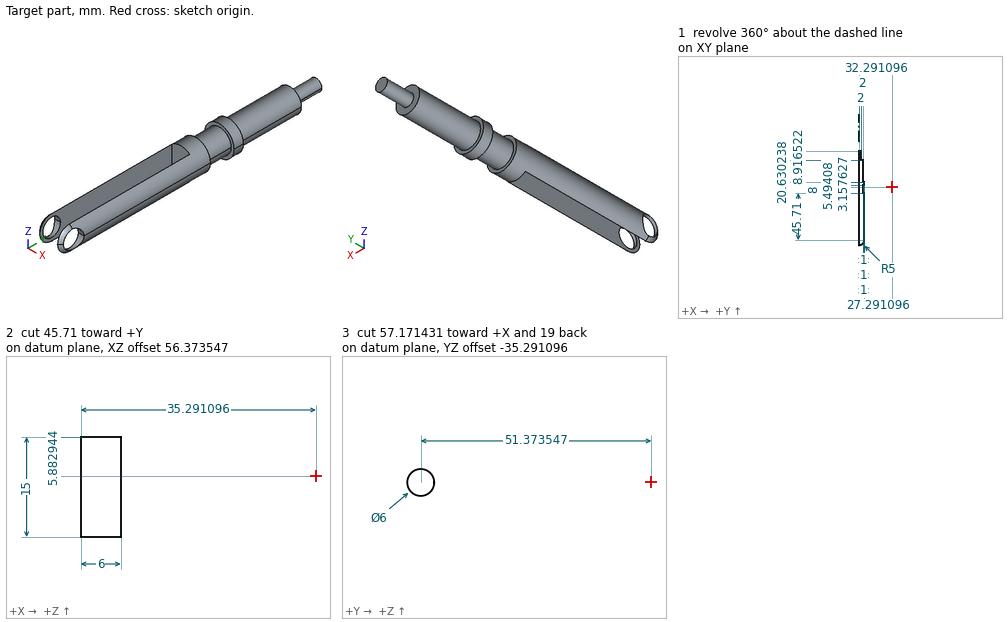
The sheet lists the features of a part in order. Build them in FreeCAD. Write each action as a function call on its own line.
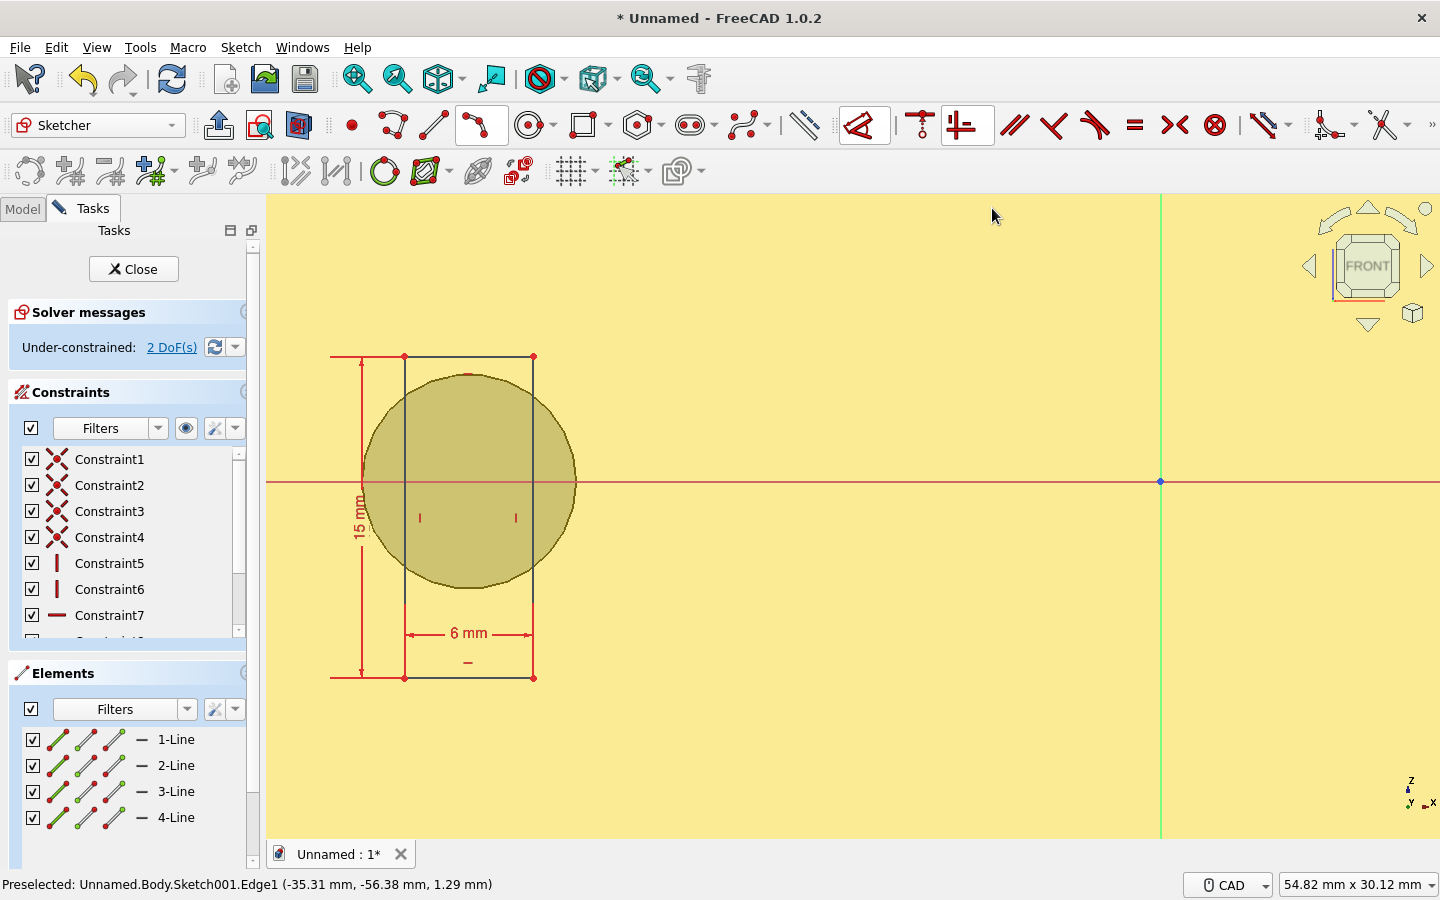
click(405, 357)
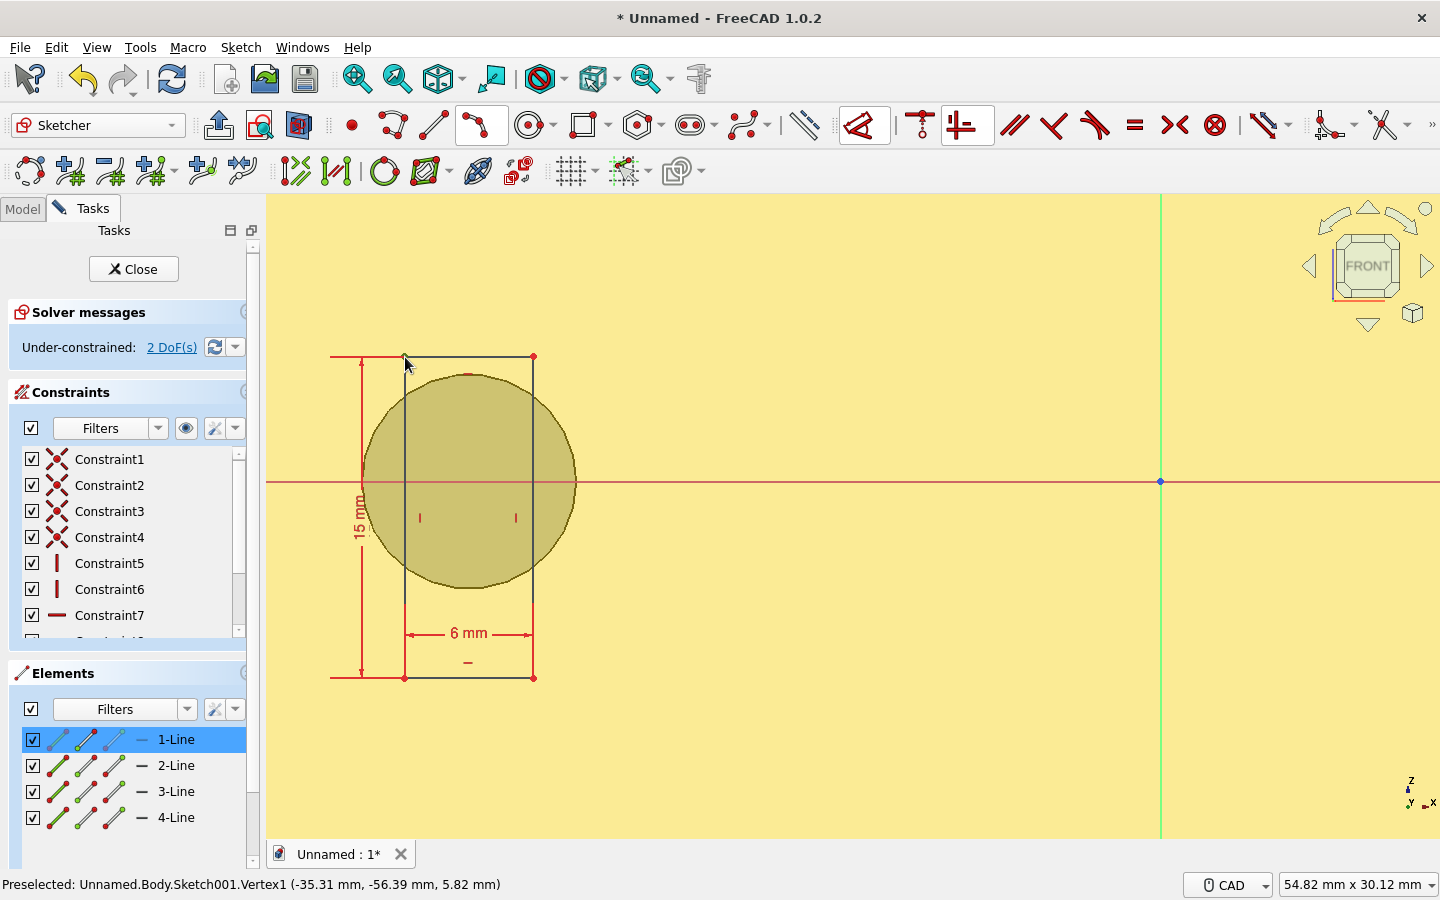
click(884, 126)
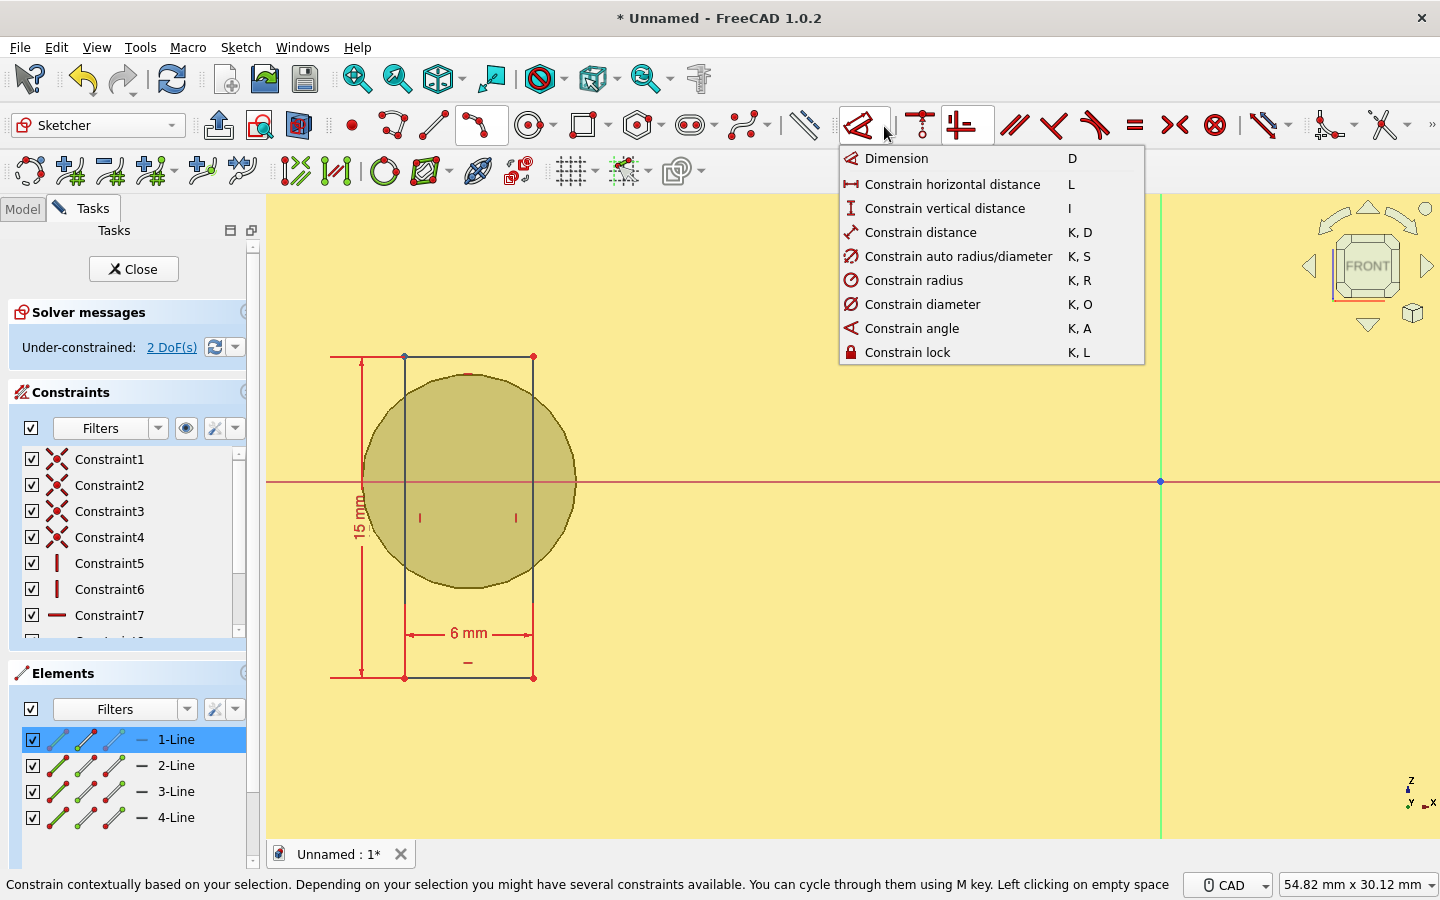
click(992, 208)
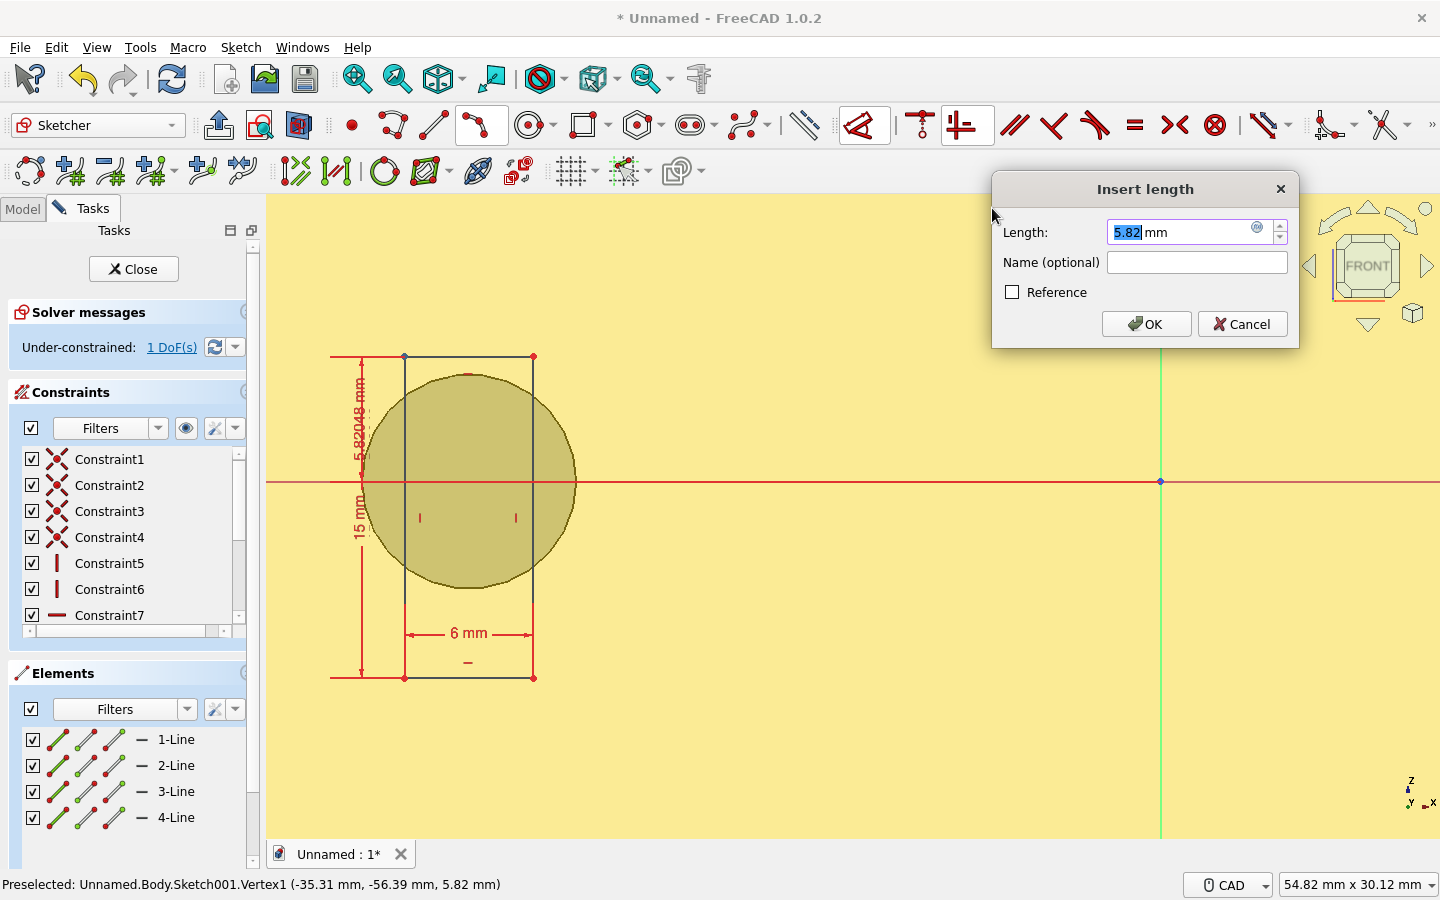
text(5.882944)
key(Return)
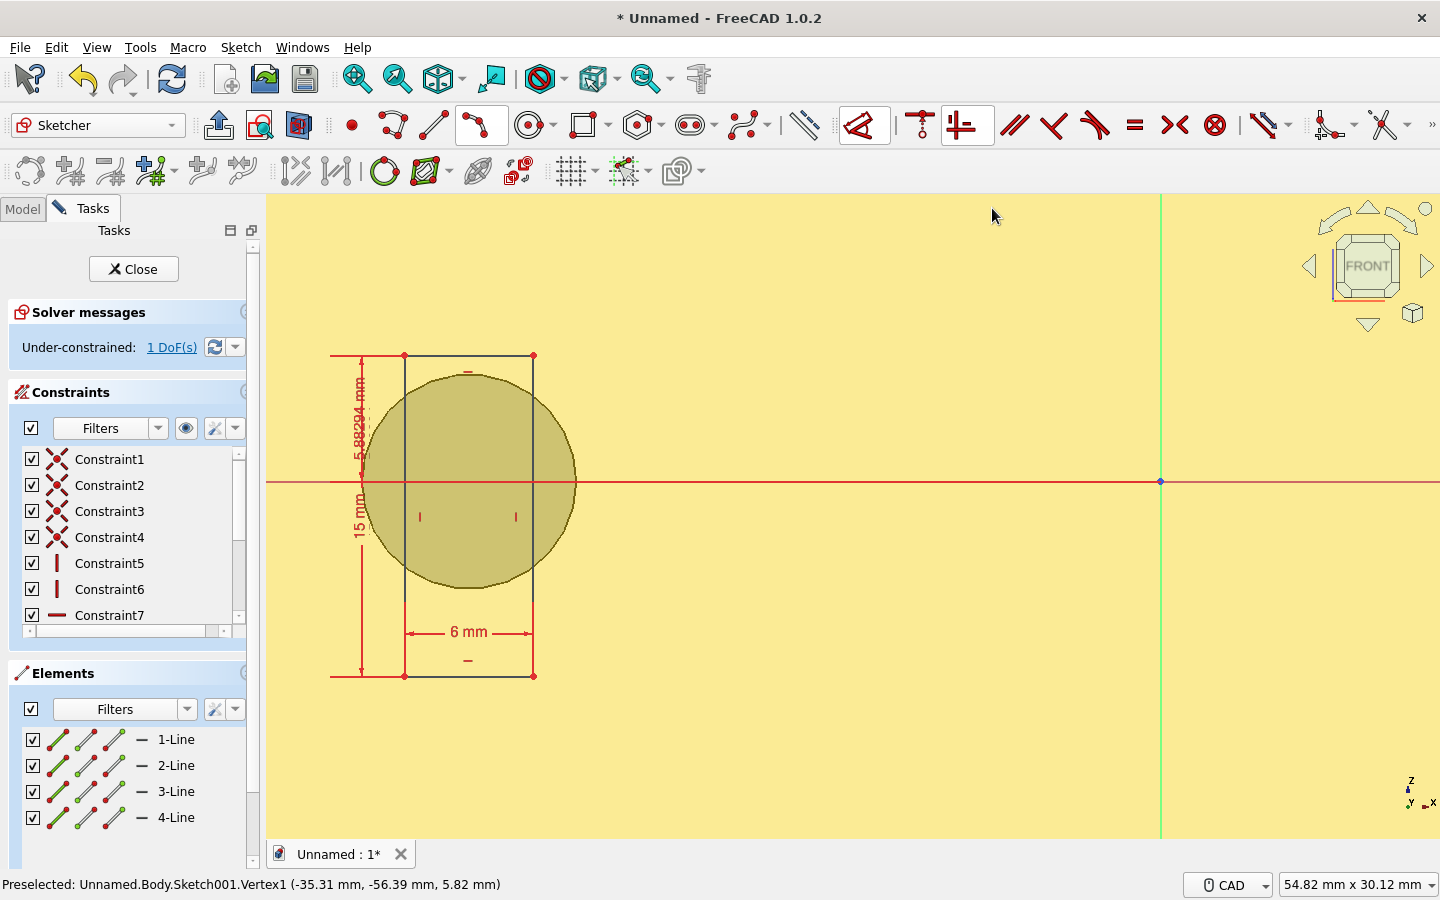
click(405, 356)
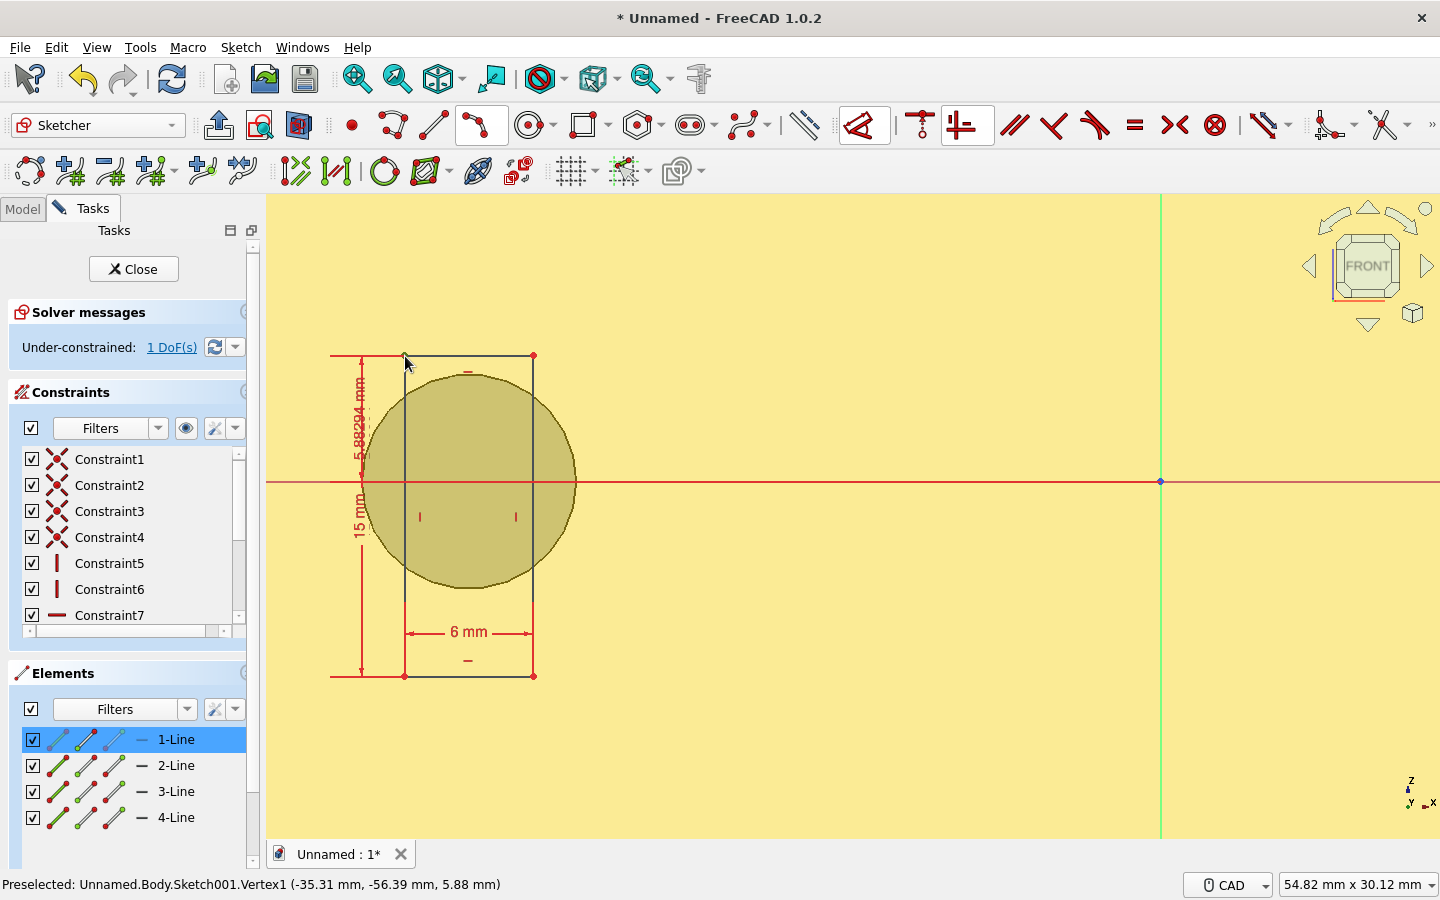
key(l)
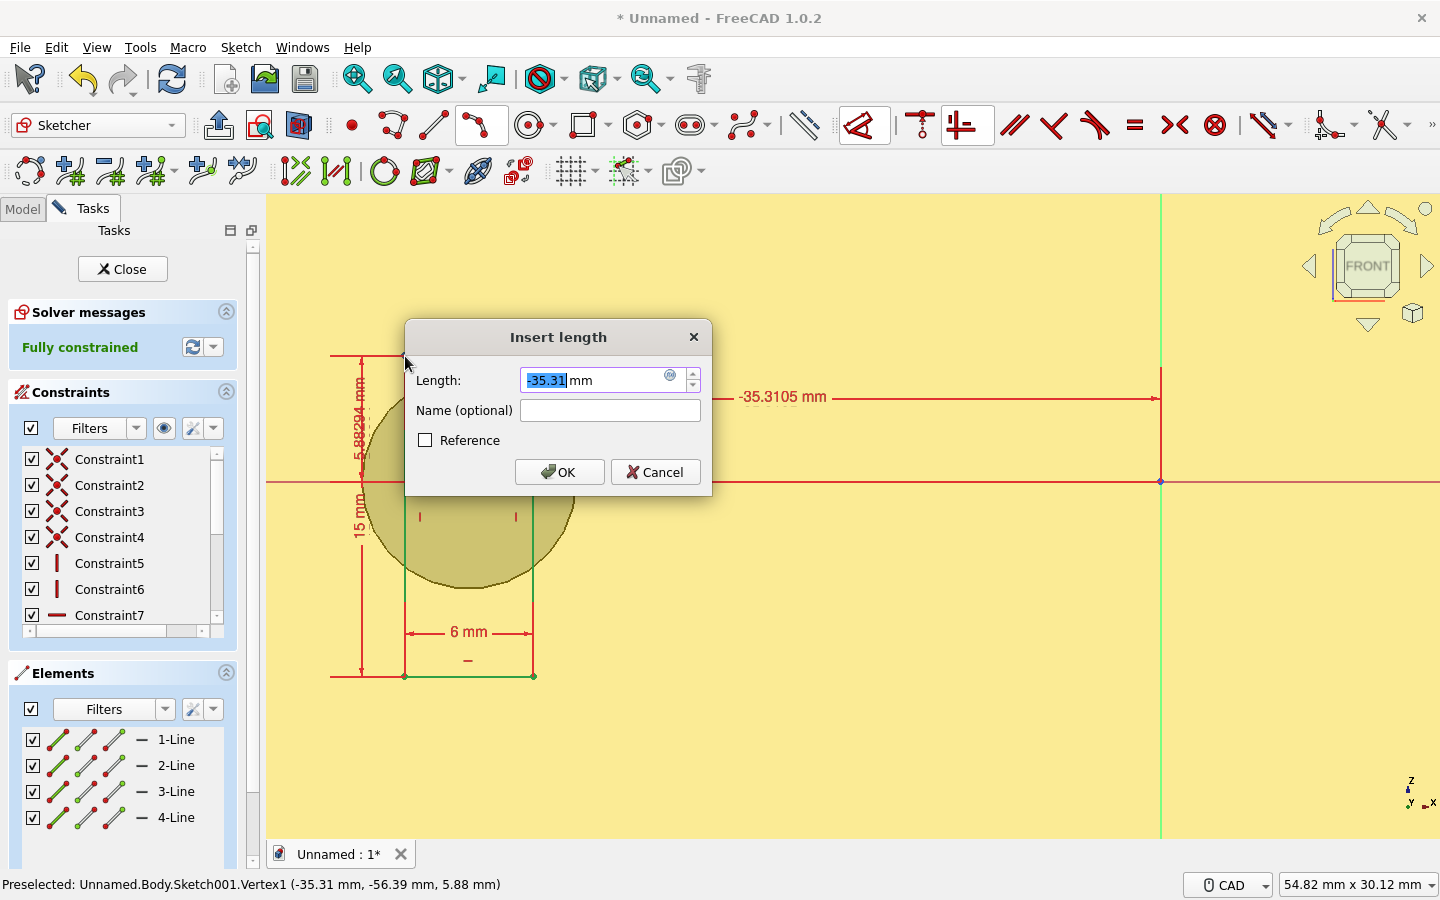
text(-35.291096)
key(Return)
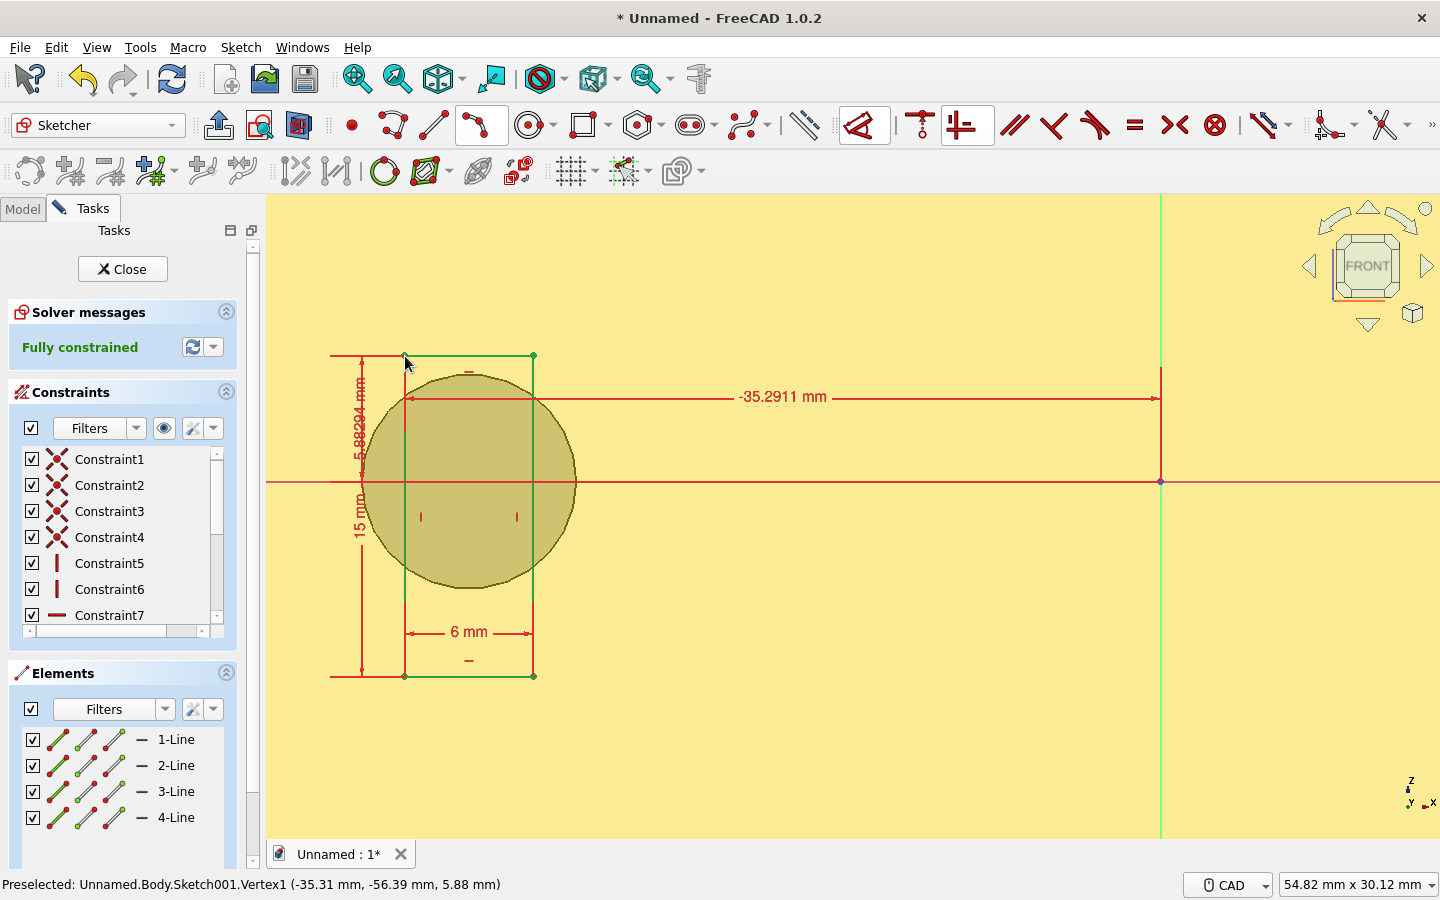
click(123, 269)